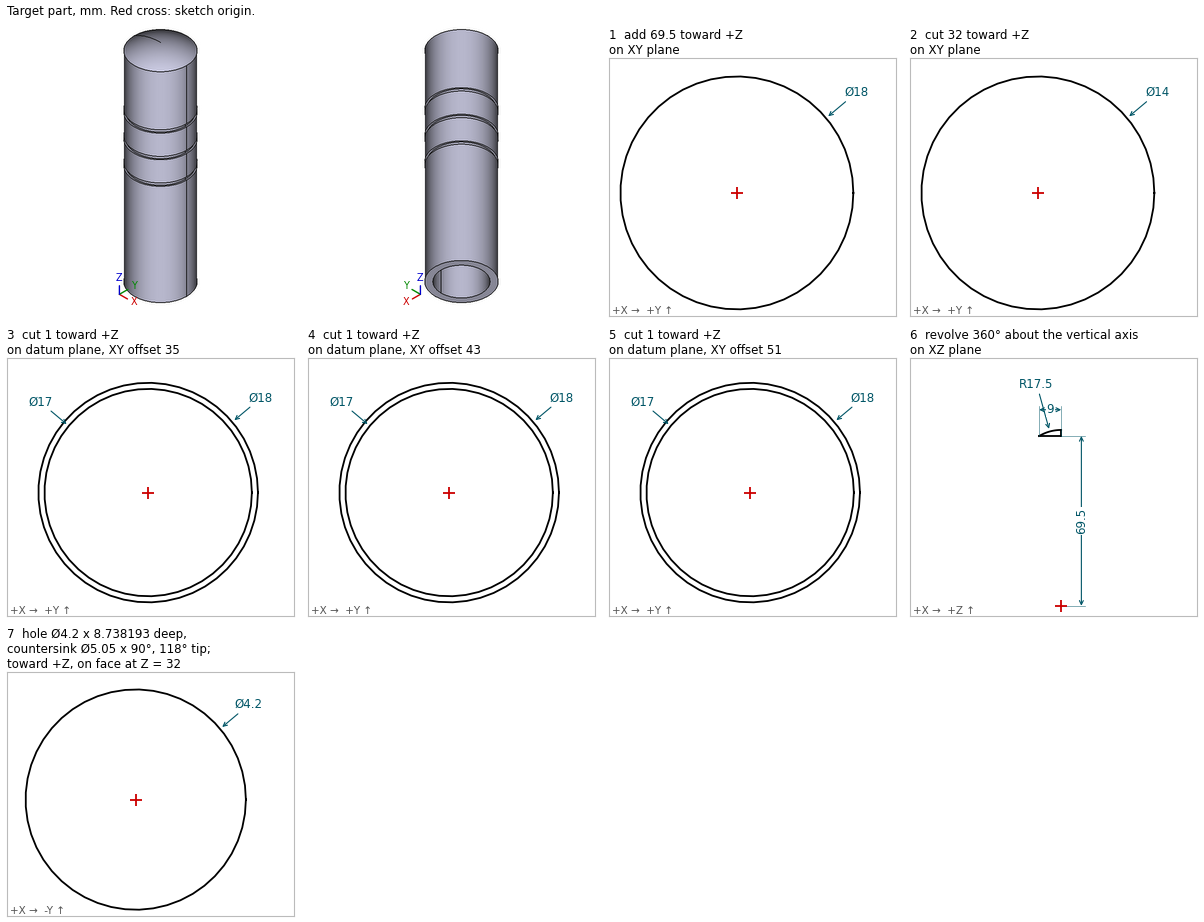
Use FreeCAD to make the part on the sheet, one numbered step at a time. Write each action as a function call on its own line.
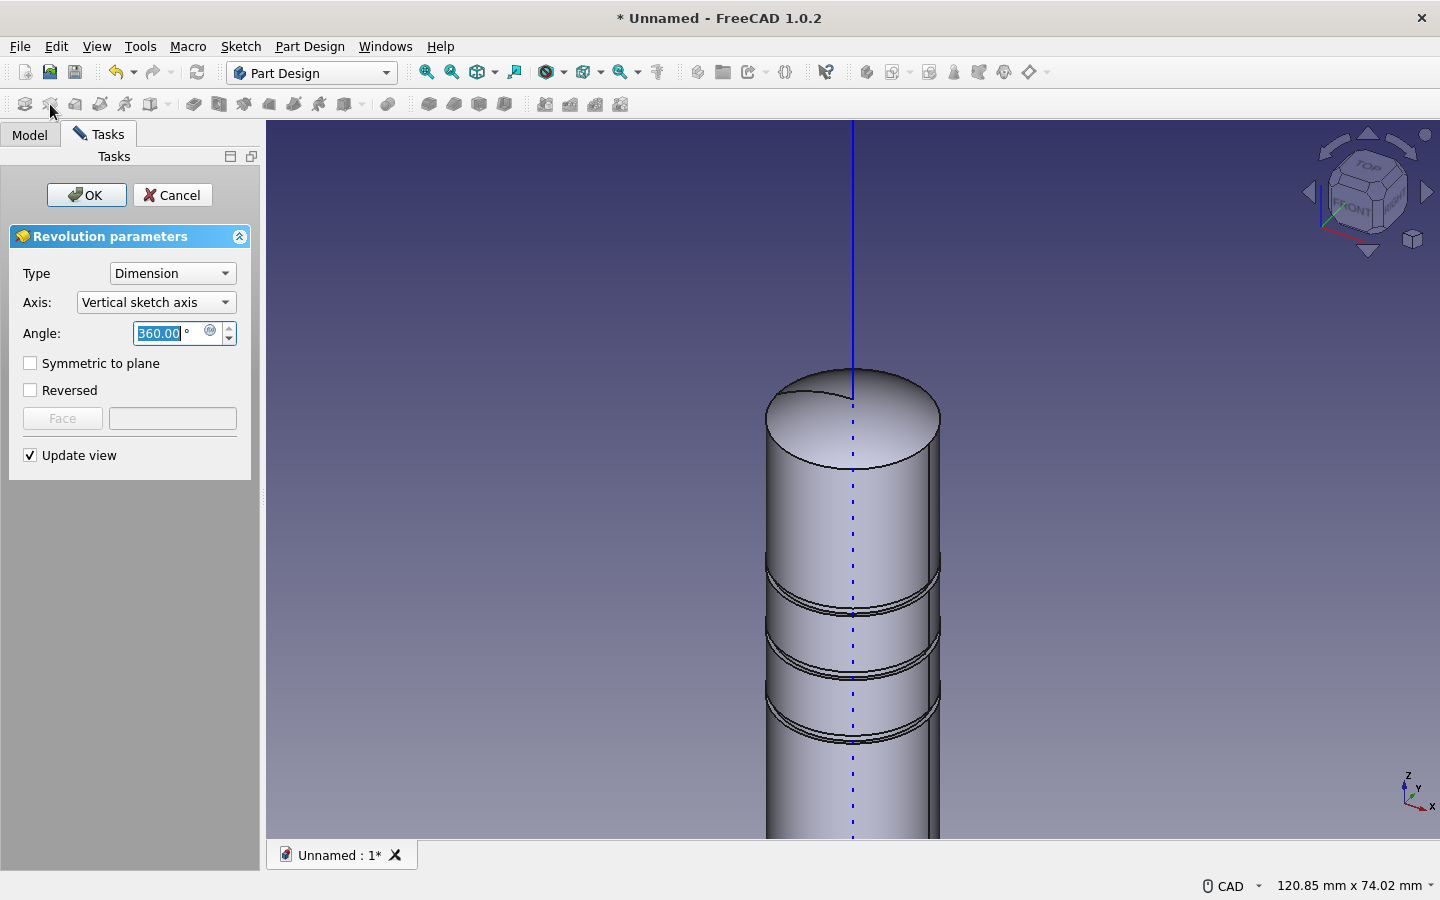
click(87, 195)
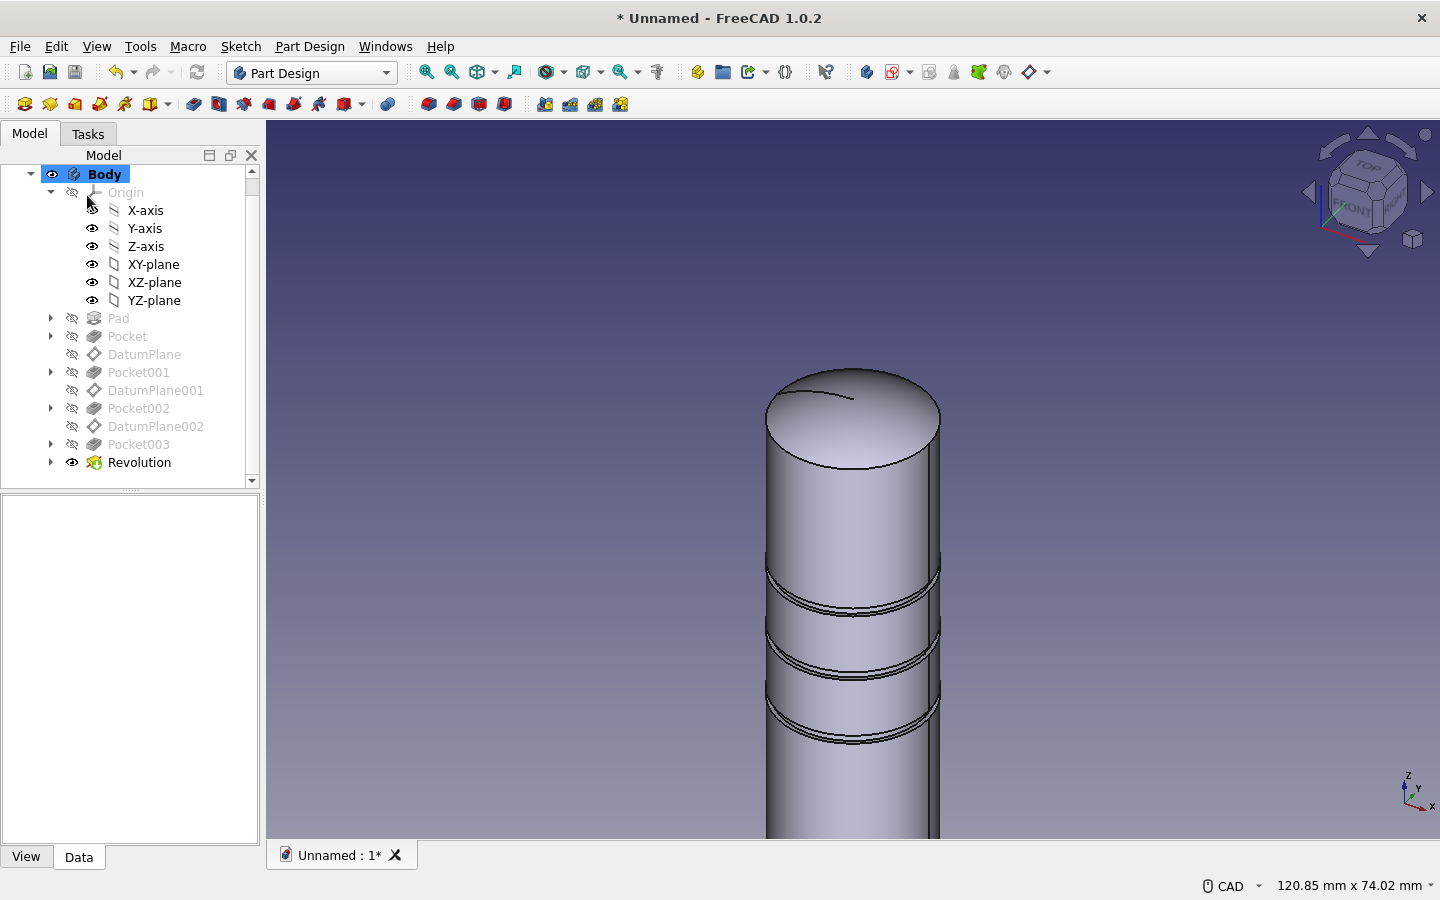
key(v)
key(f)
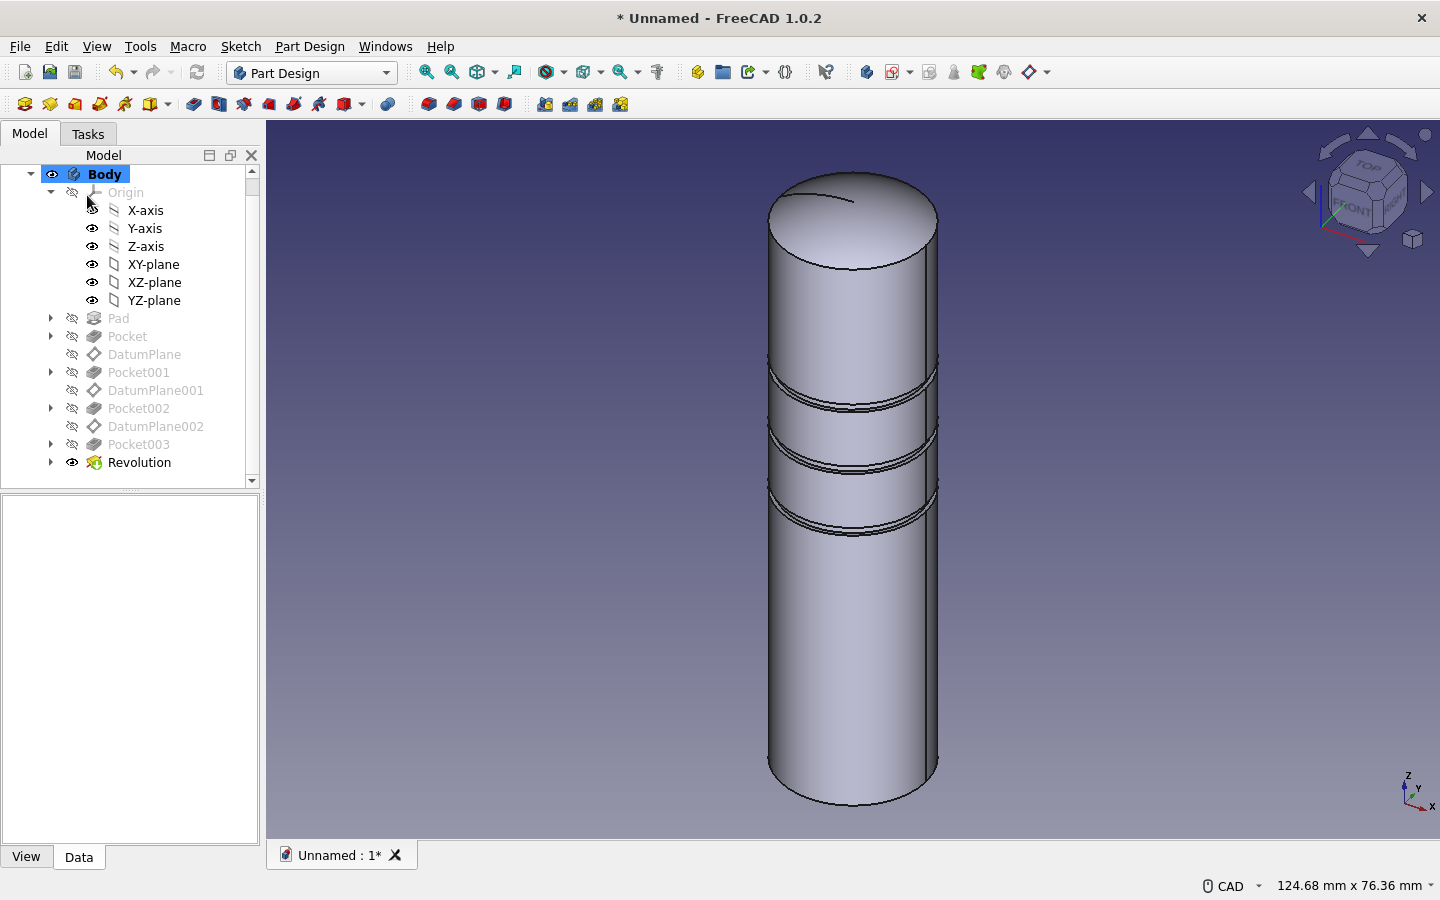
key(5)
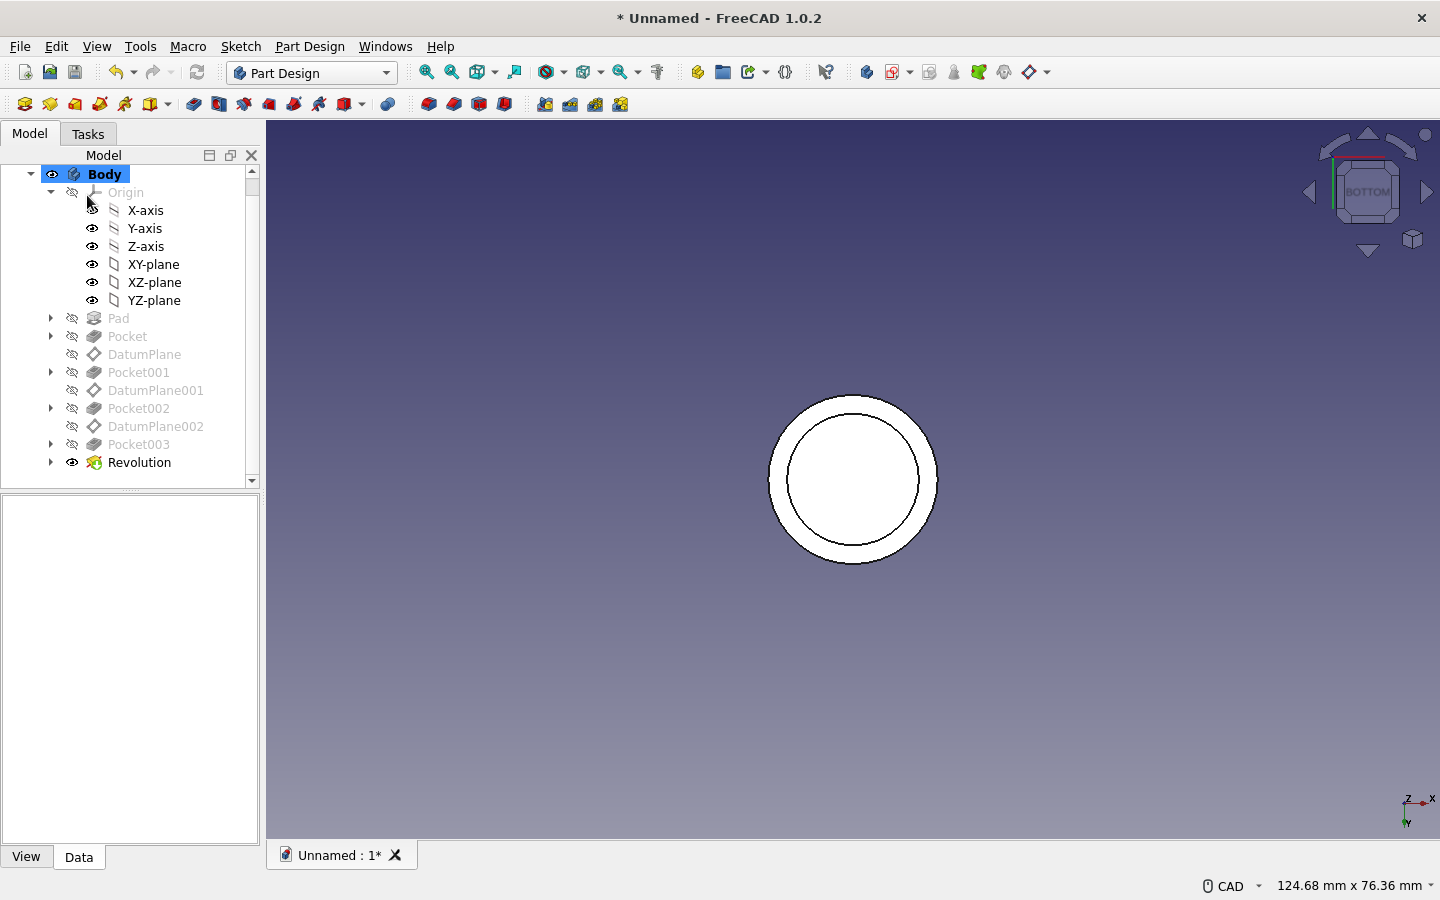
key(v)
key(f)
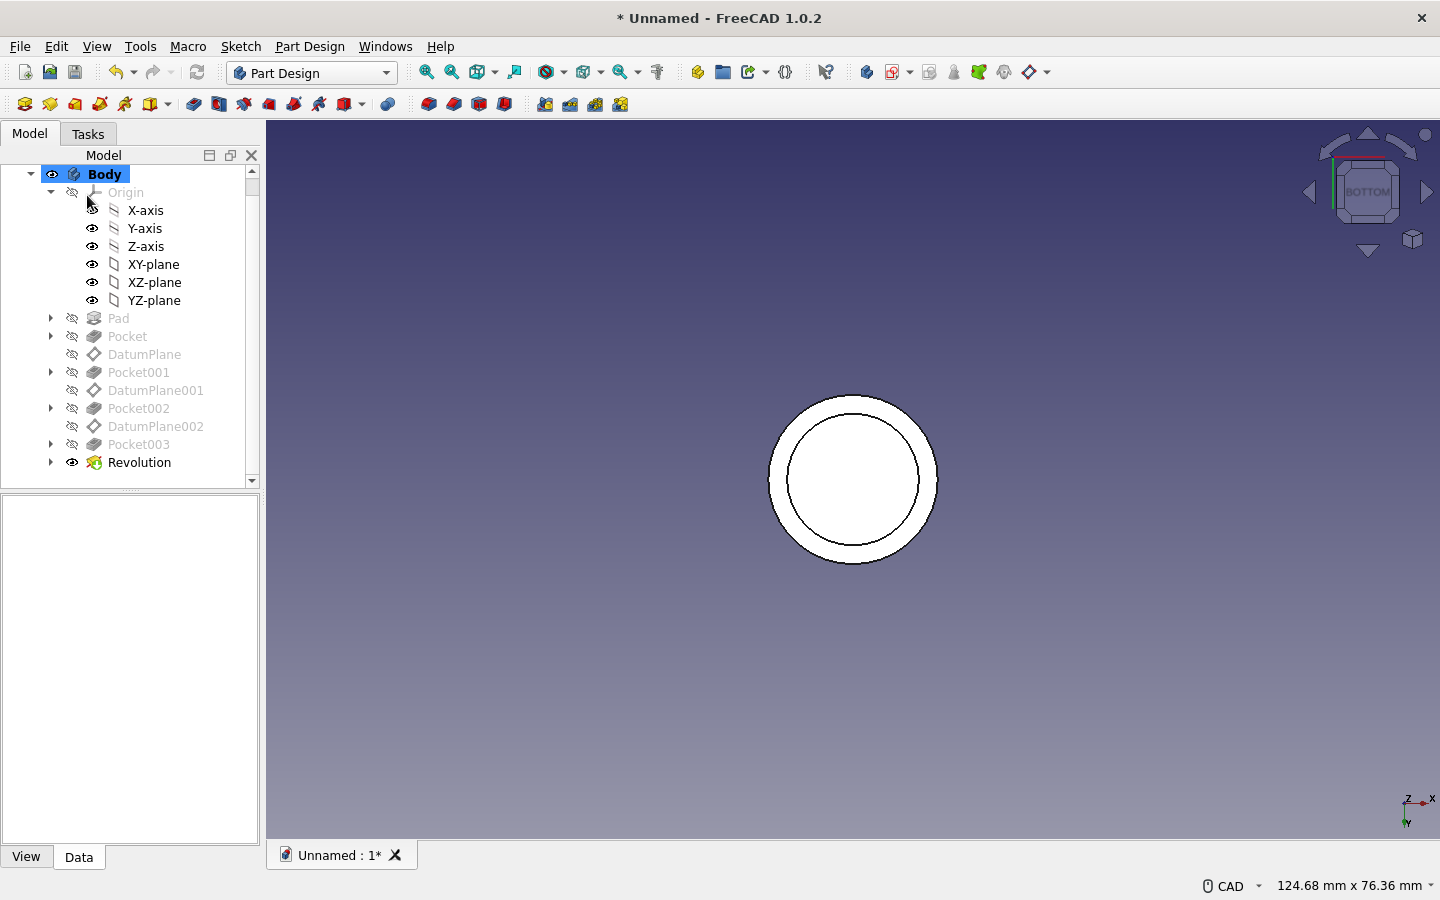
click(853, 478)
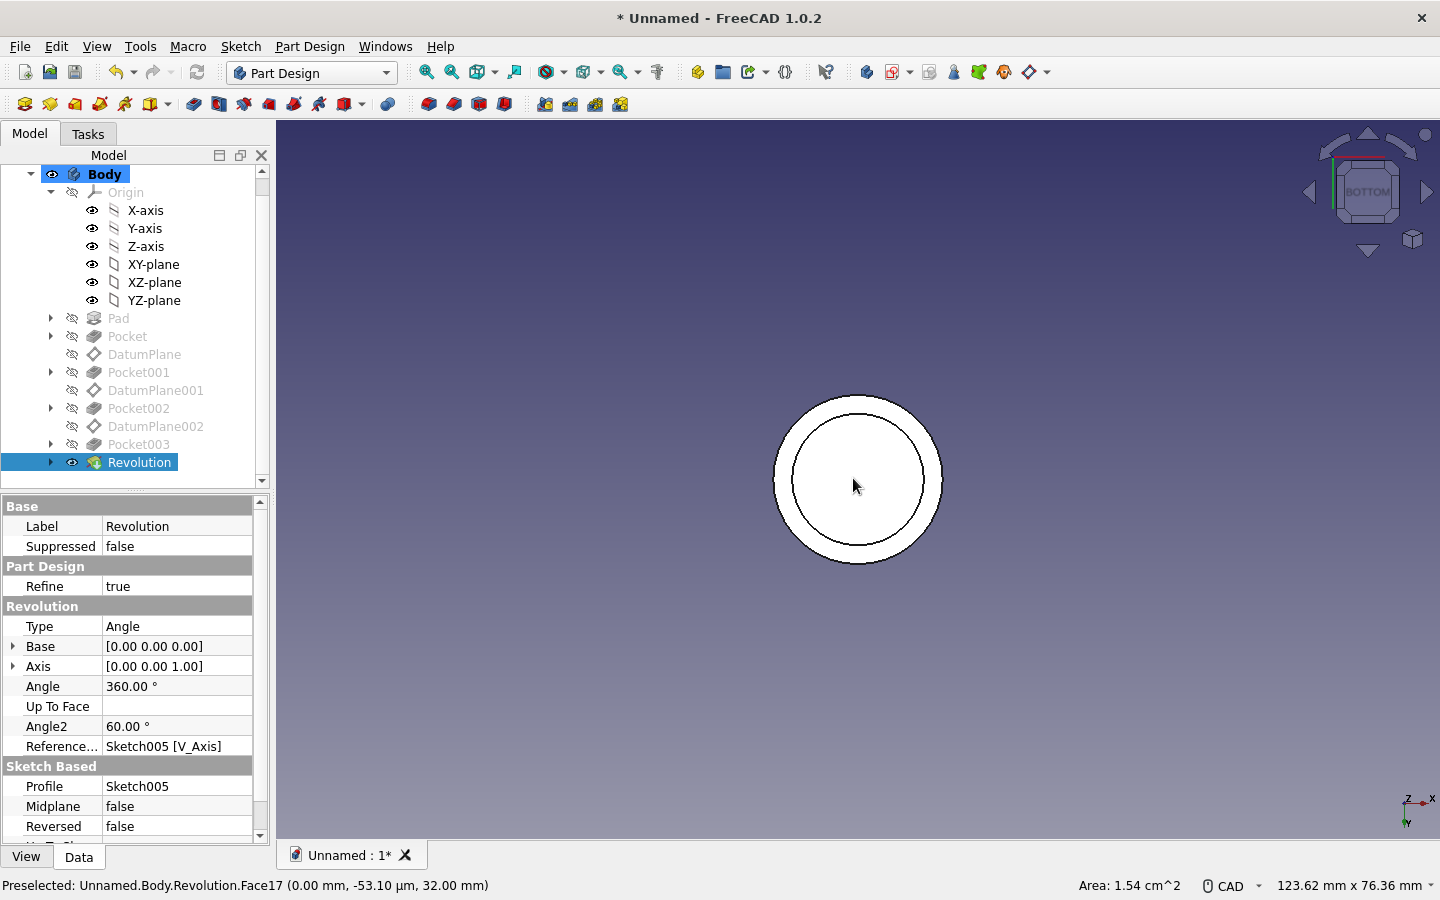
click(892, 72)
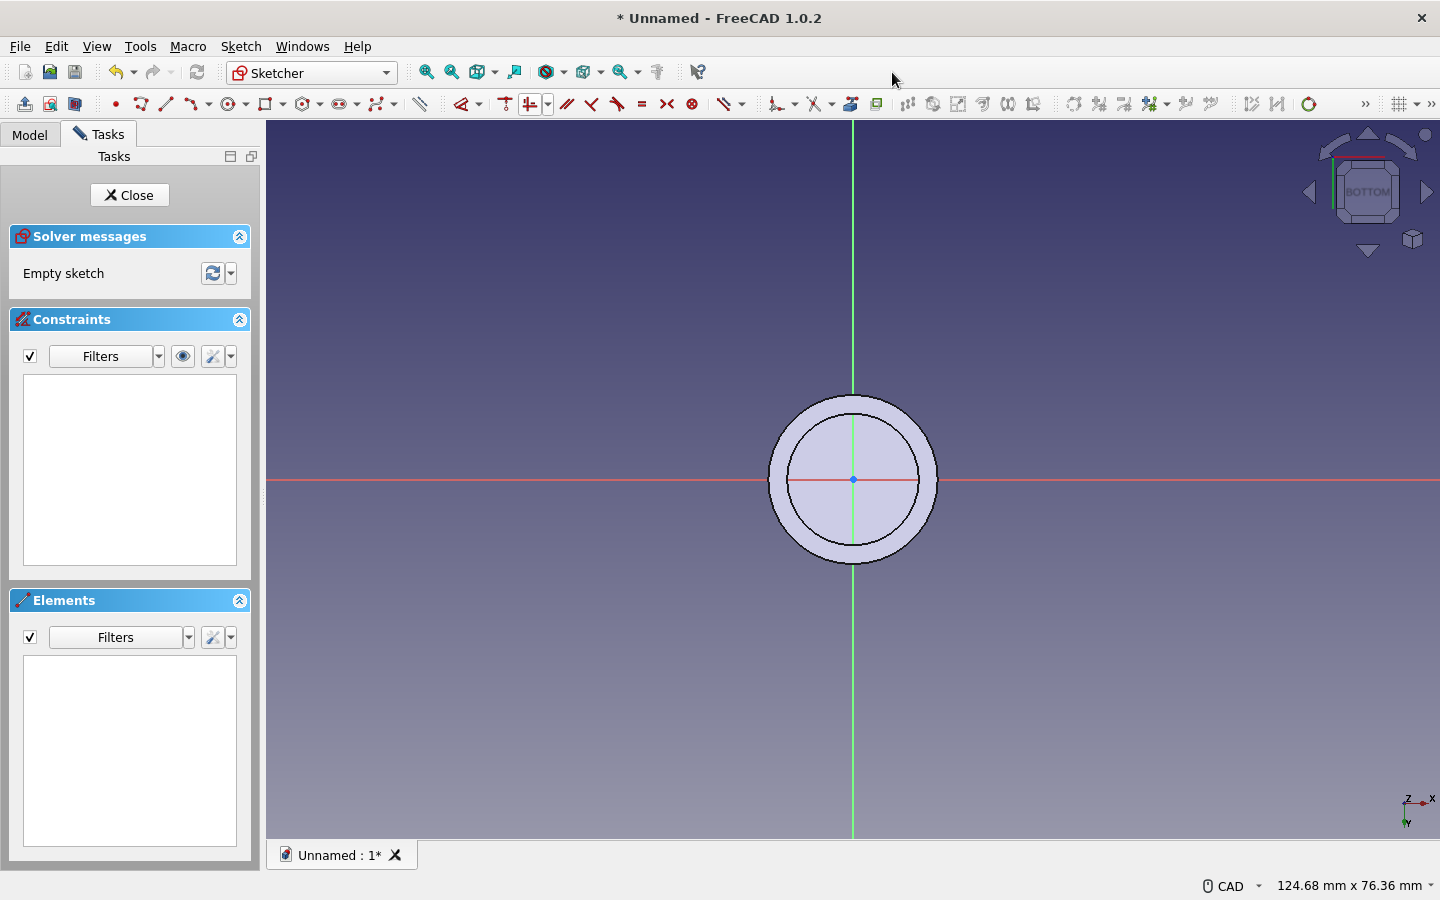
click(75, 104)